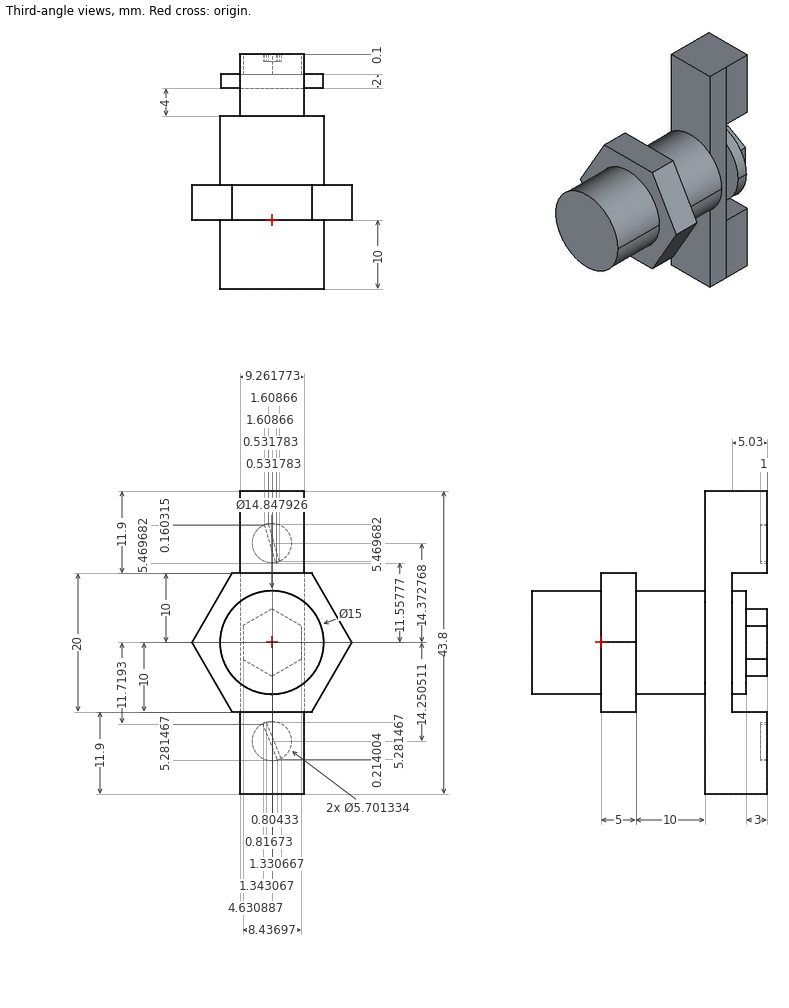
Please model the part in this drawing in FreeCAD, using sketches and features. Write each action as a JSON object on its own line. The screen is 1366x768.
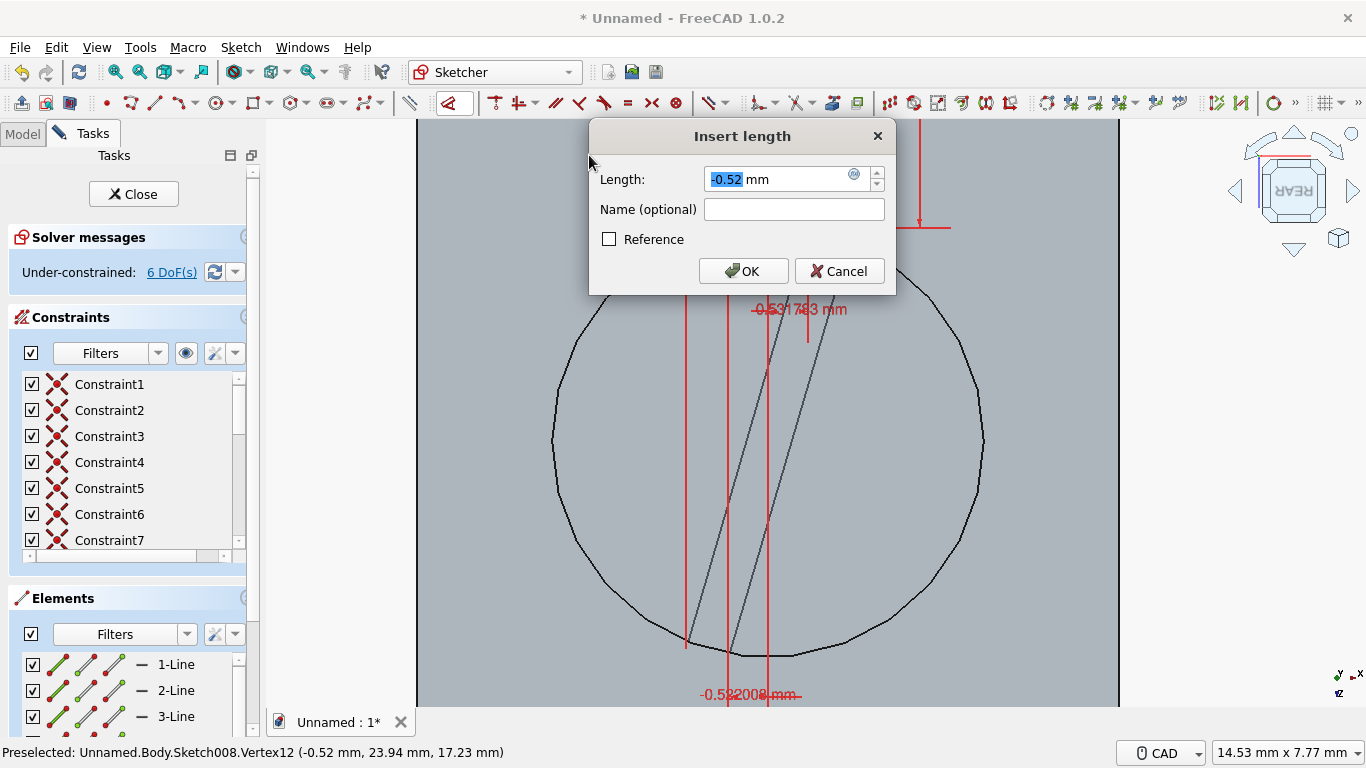
{"action": "type", "text": "-0.531783"}
{"action": "key", "text": "Return"}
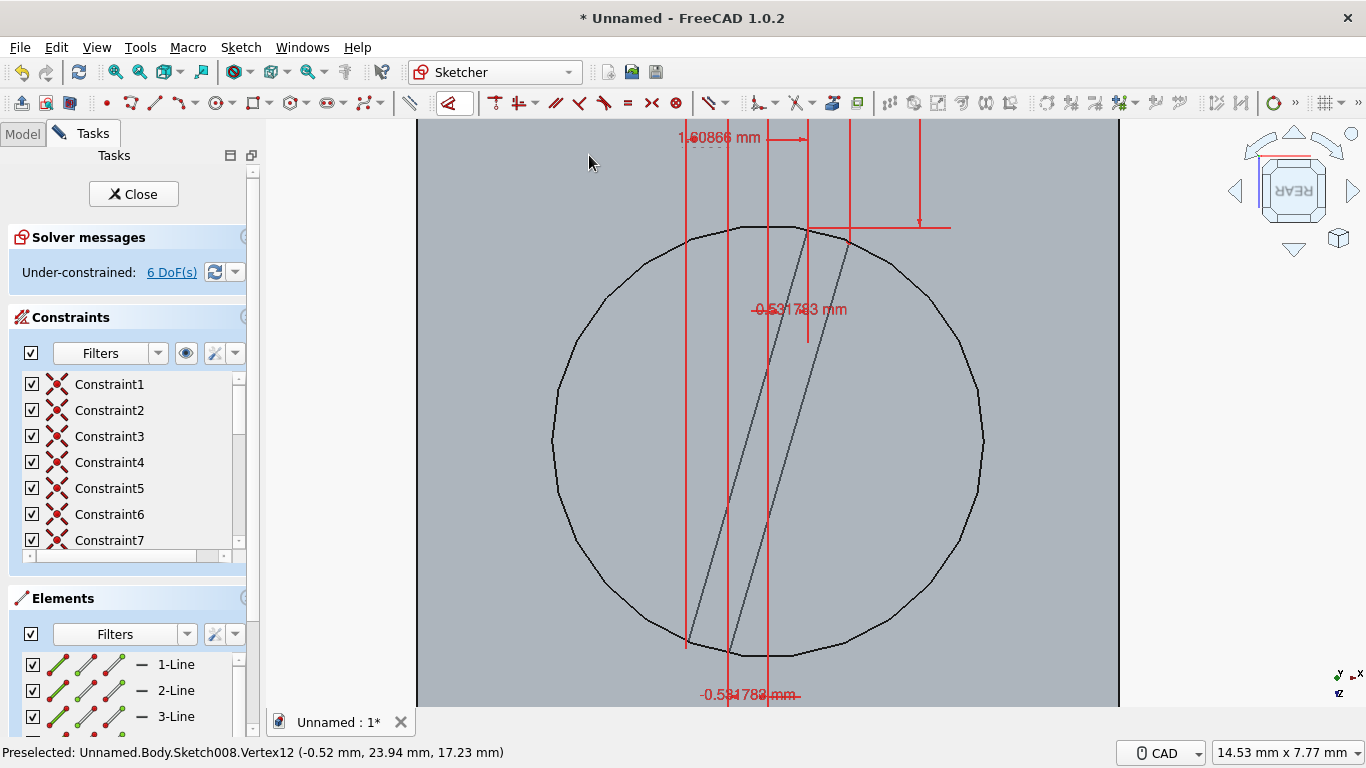
{"action": "scroll", "coordinate": [744, 578], "scroll_direction": "down", "scroll_amount": 10}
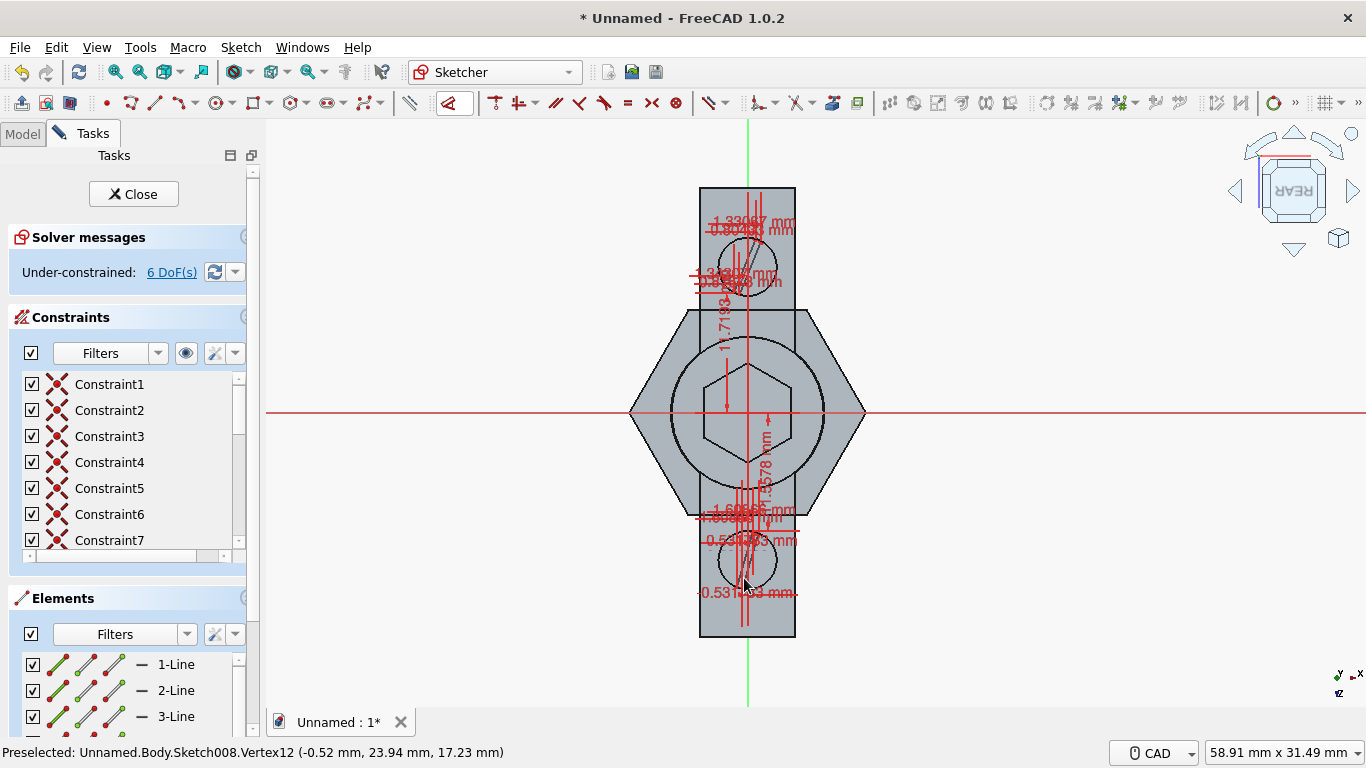
{"action": "scroll", "coordinate": [746, 279], "scroll_direction": "up", "scroll_amount": 11}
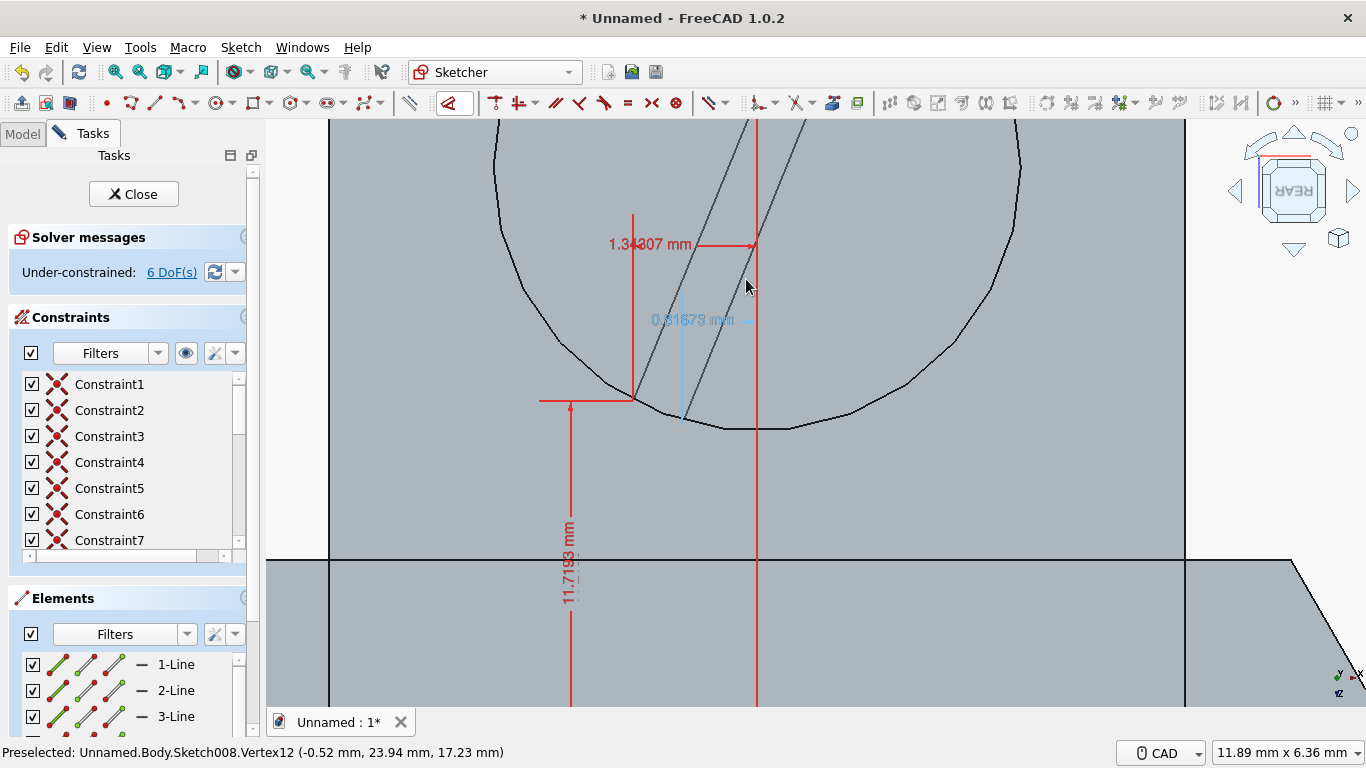
{"action": "left_click", "coordinate": [741, 279]}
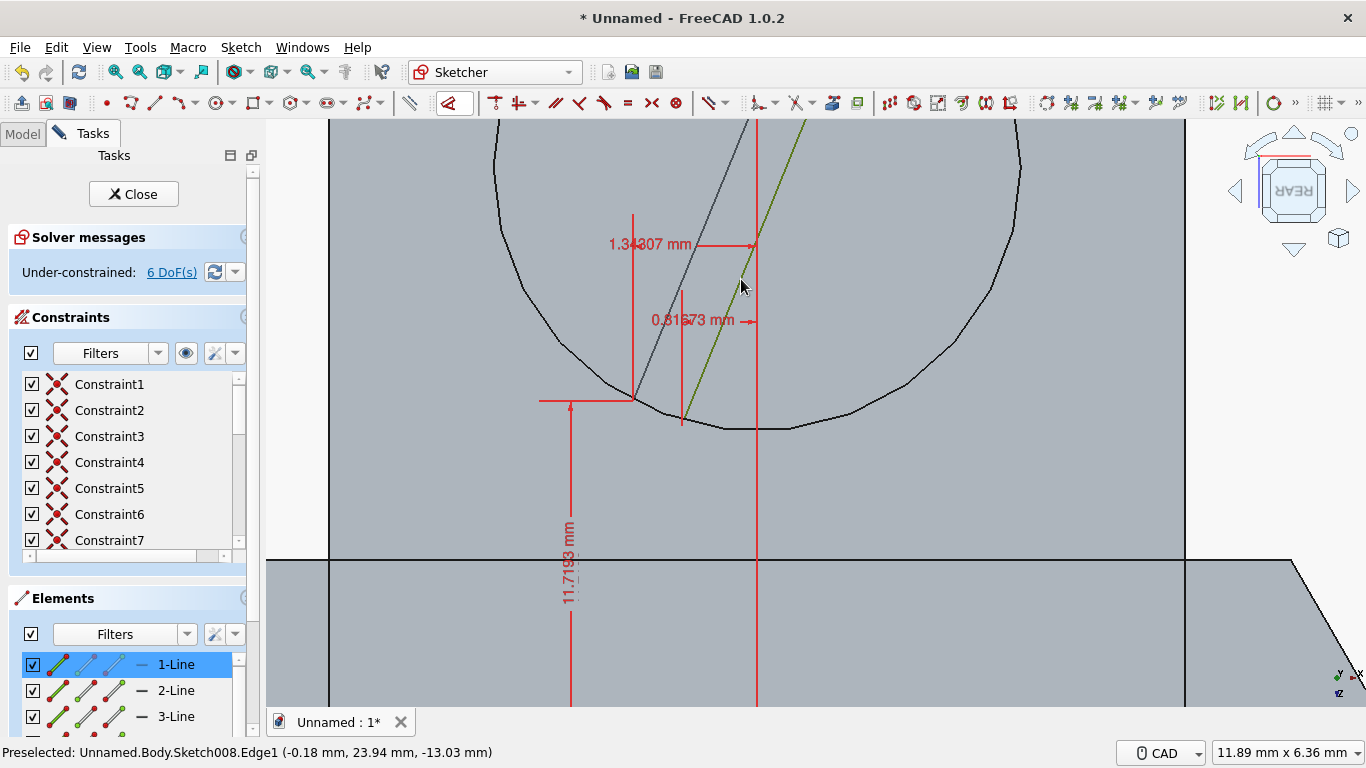
{"action": "left_click", "coordinate": [468, 104]}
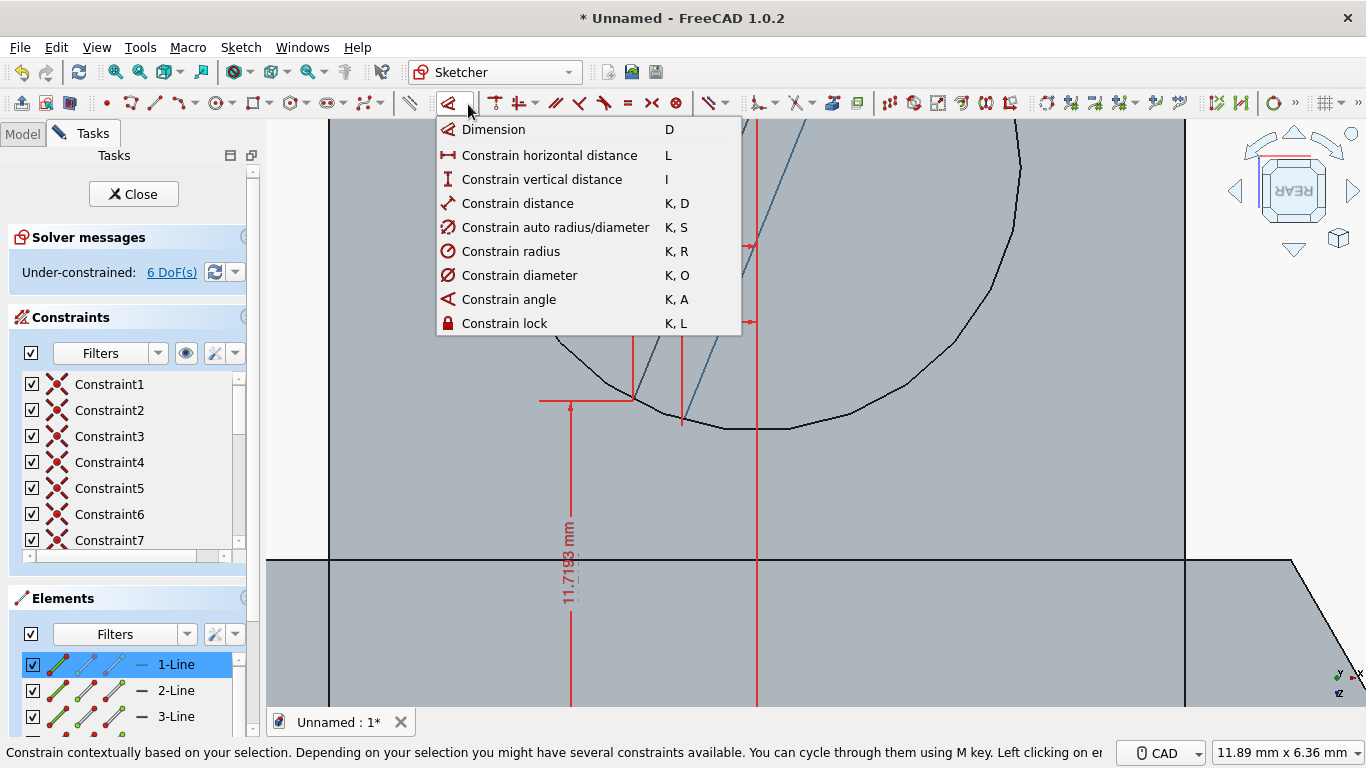
{"action": "left_click", "coordinate": [589, 179]}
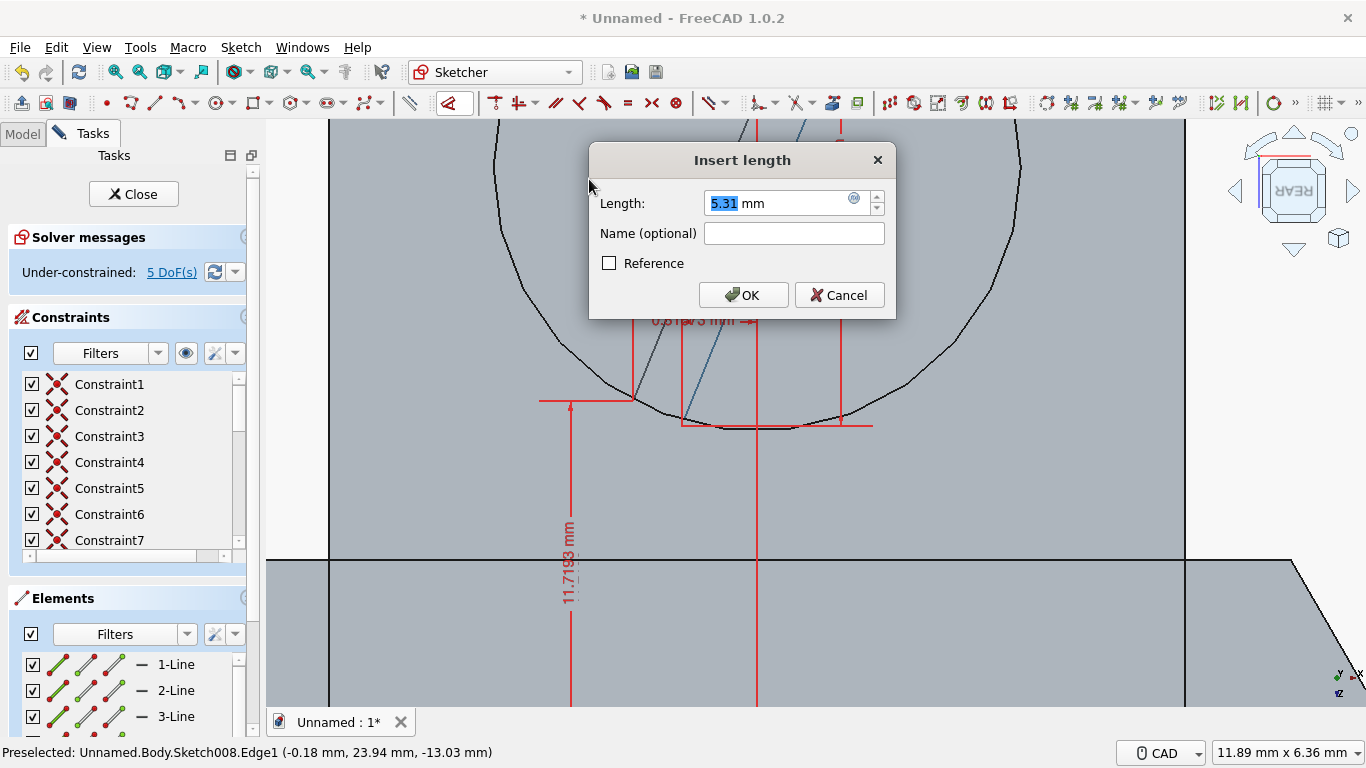
{"action": "type", "text": "5.281467"}
{"action": "key", "text": "Return"}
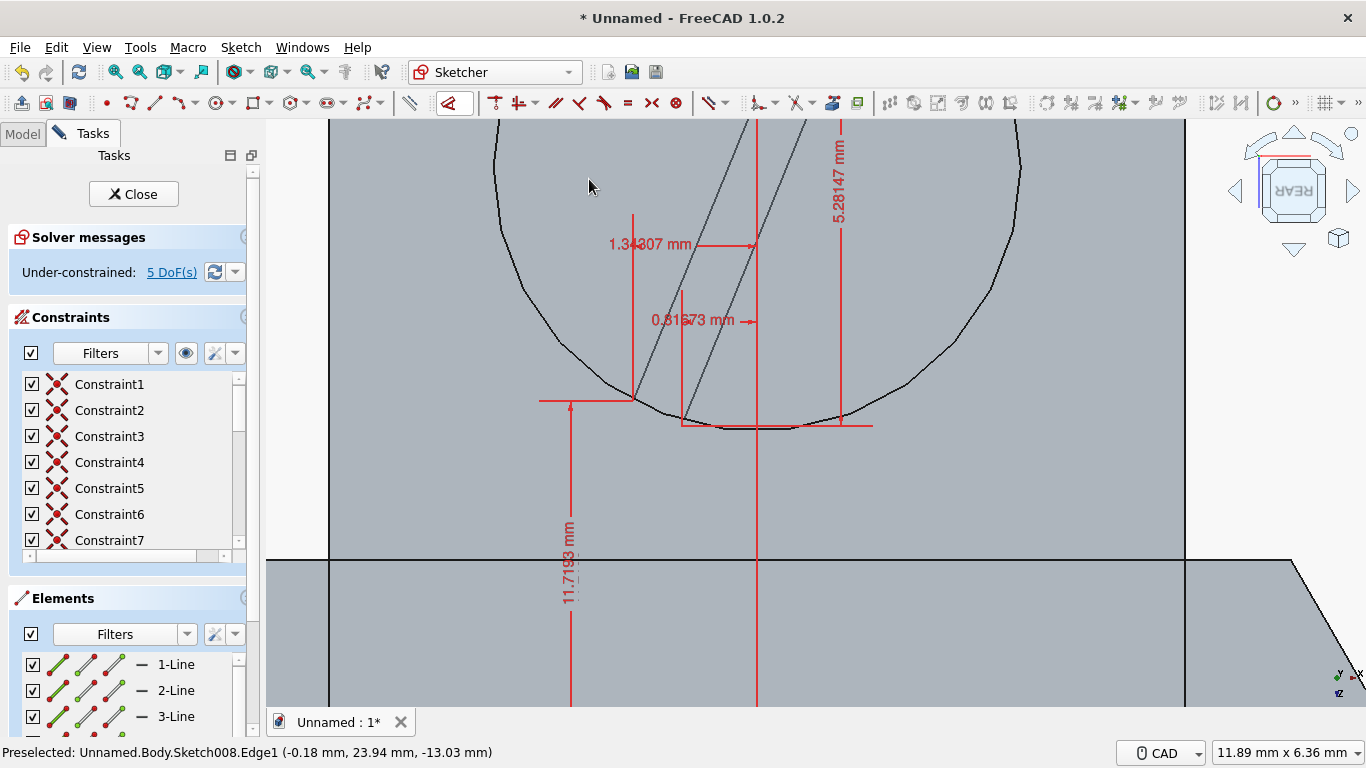
{"action": "scroll", "coordinate": [746, 278], "scroll_direction": "down", "scroll_amount": 11}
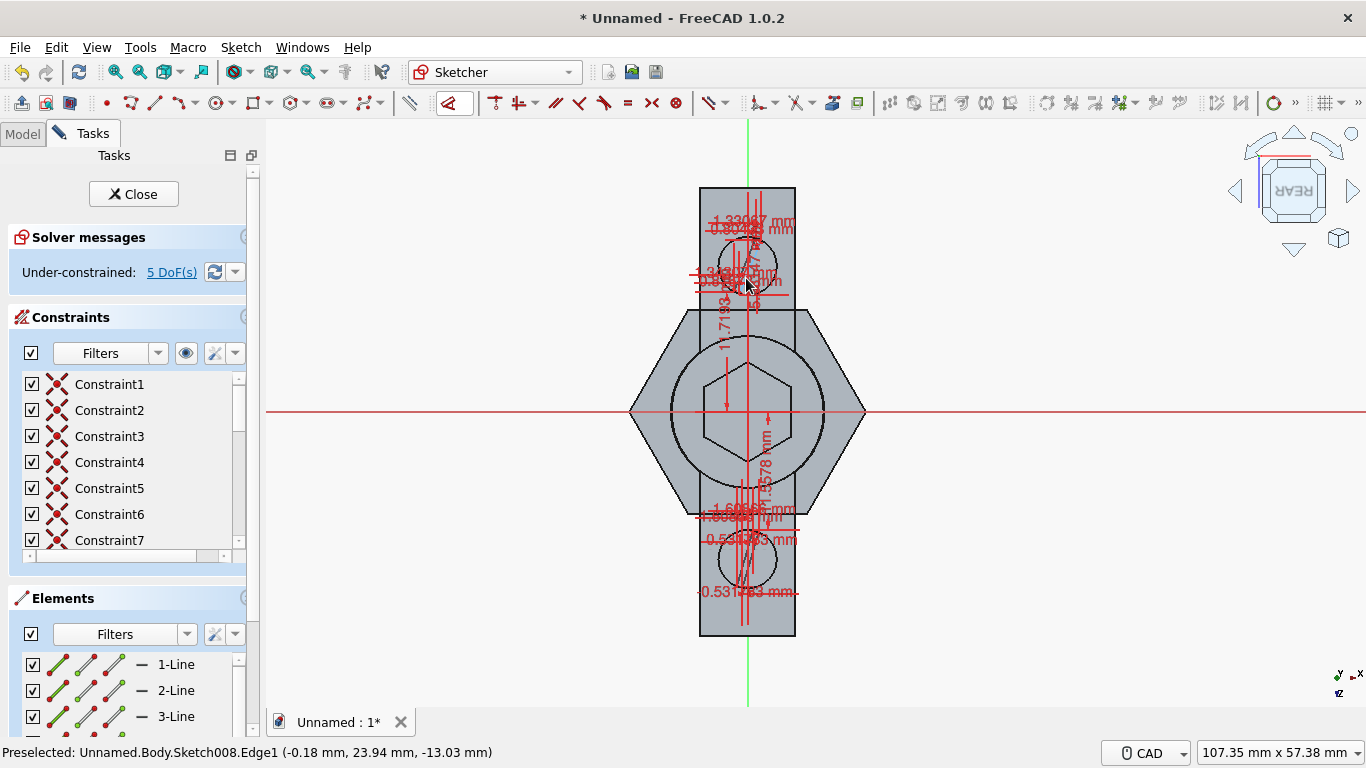
{"action": "scroll", "coordinate": [760, 240], "scroll_direction": "up", "scroll_amount": 15}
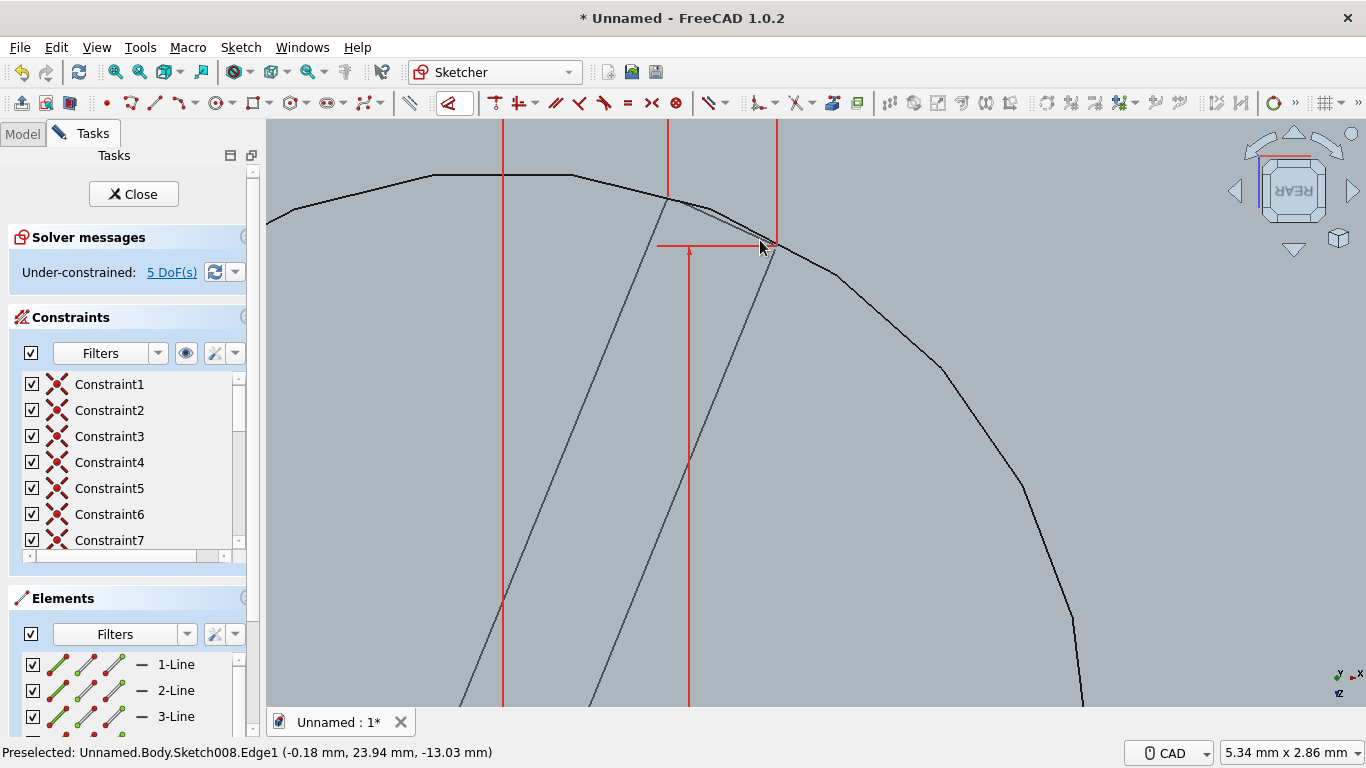
{"action": "left_click", "coordinate": [744, 231]}